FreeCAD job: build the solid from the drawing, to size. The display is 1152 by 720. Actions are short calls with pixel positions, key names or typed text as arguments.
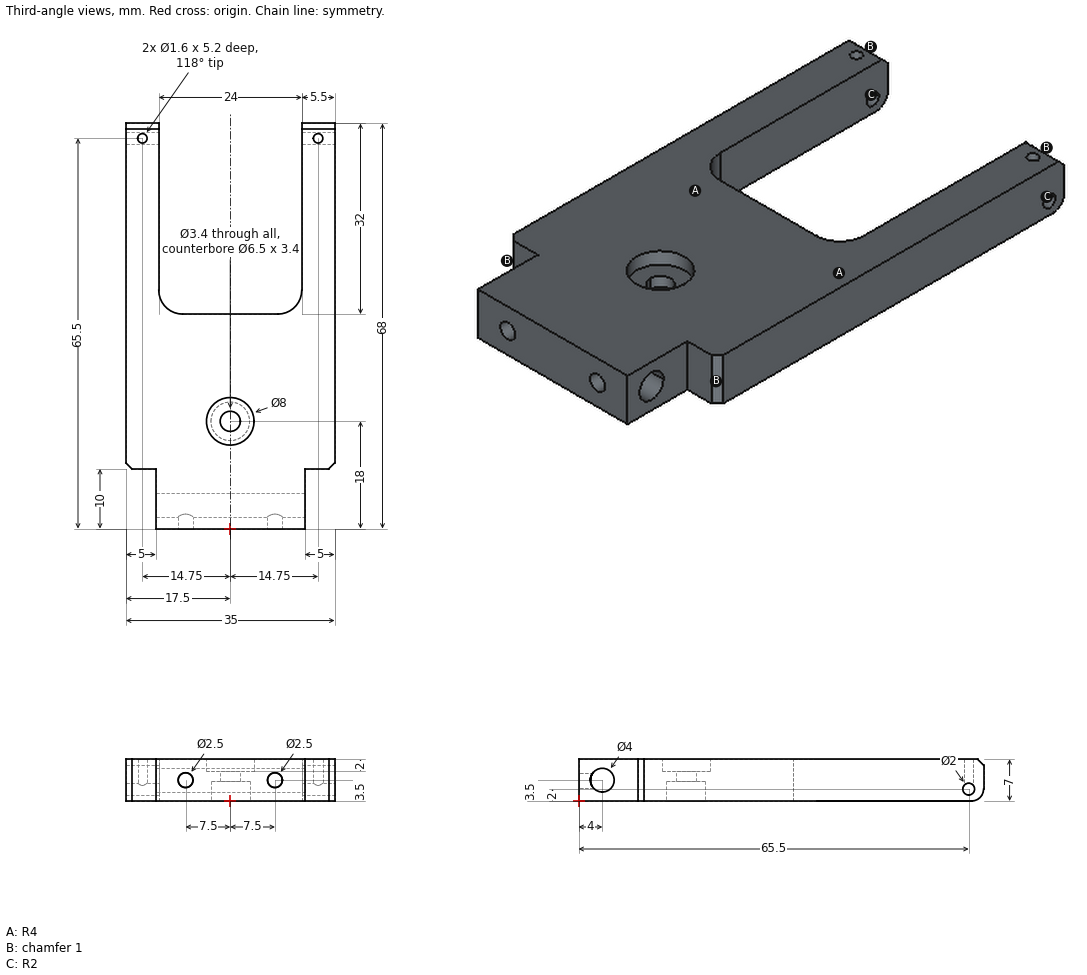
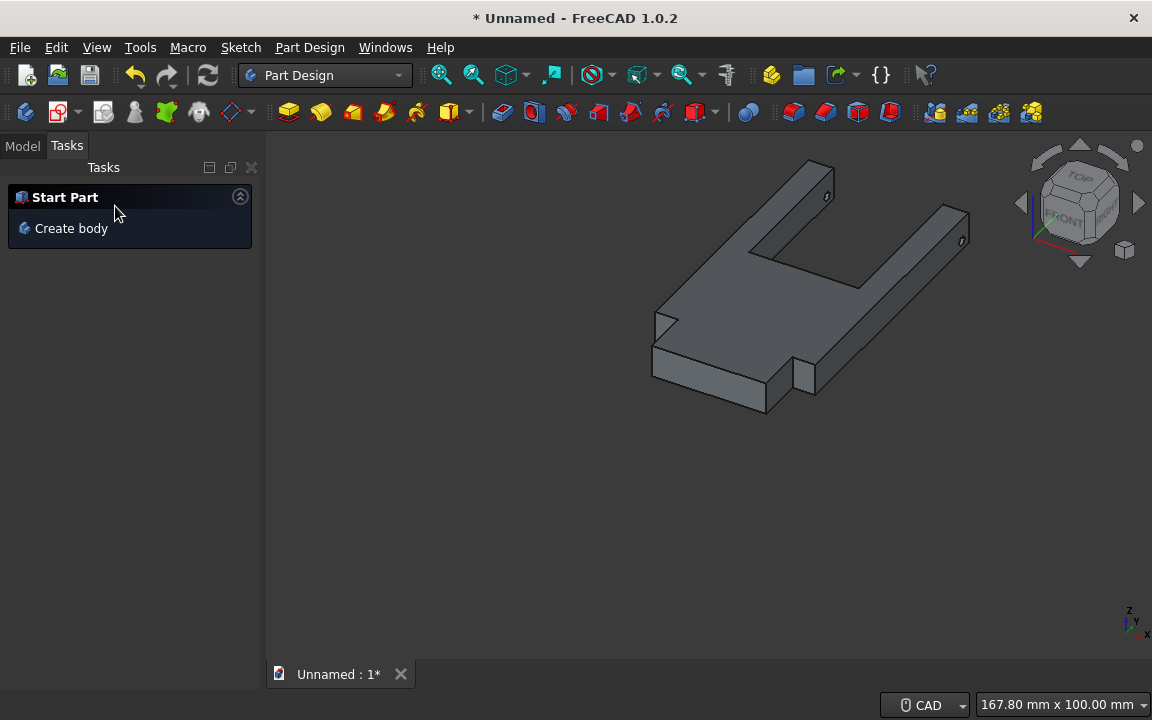
click(783, 381)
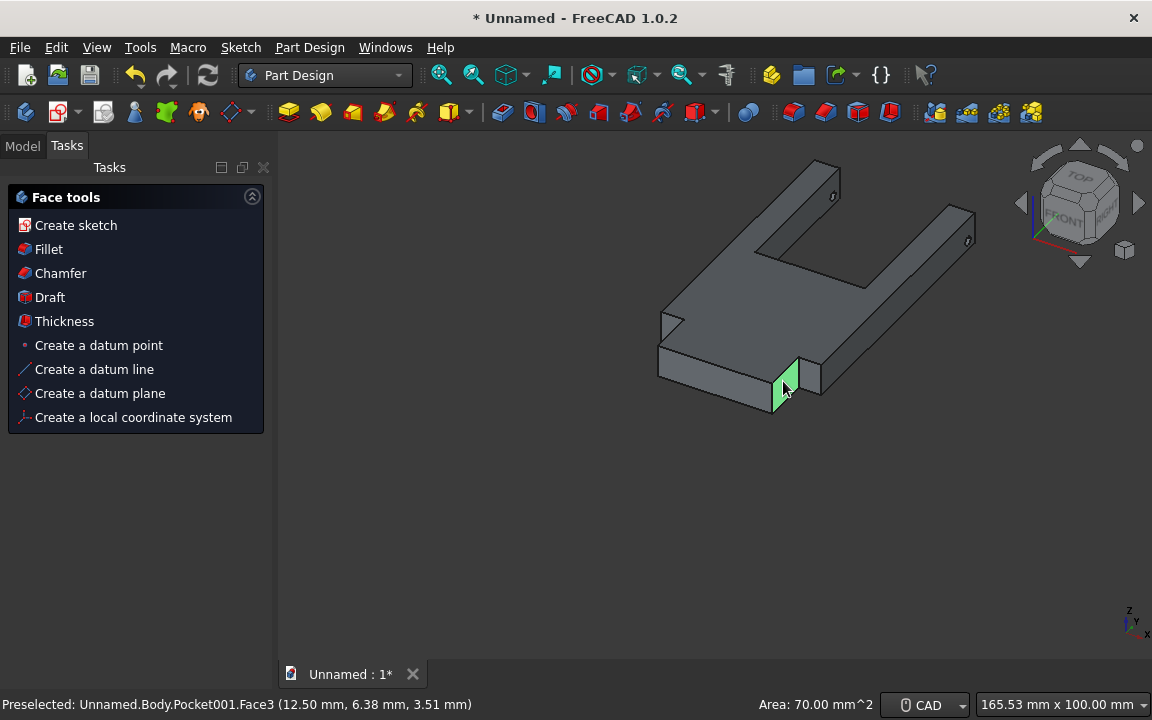
click(58, 112)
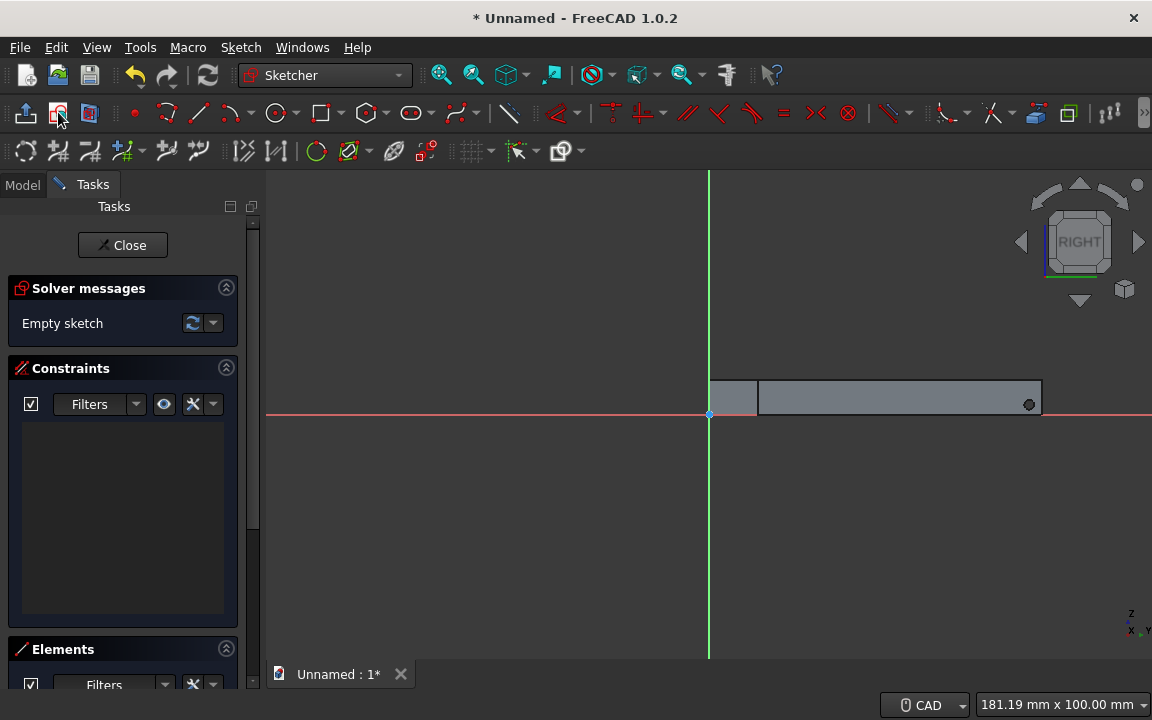
scroll(732, 400, up, 12)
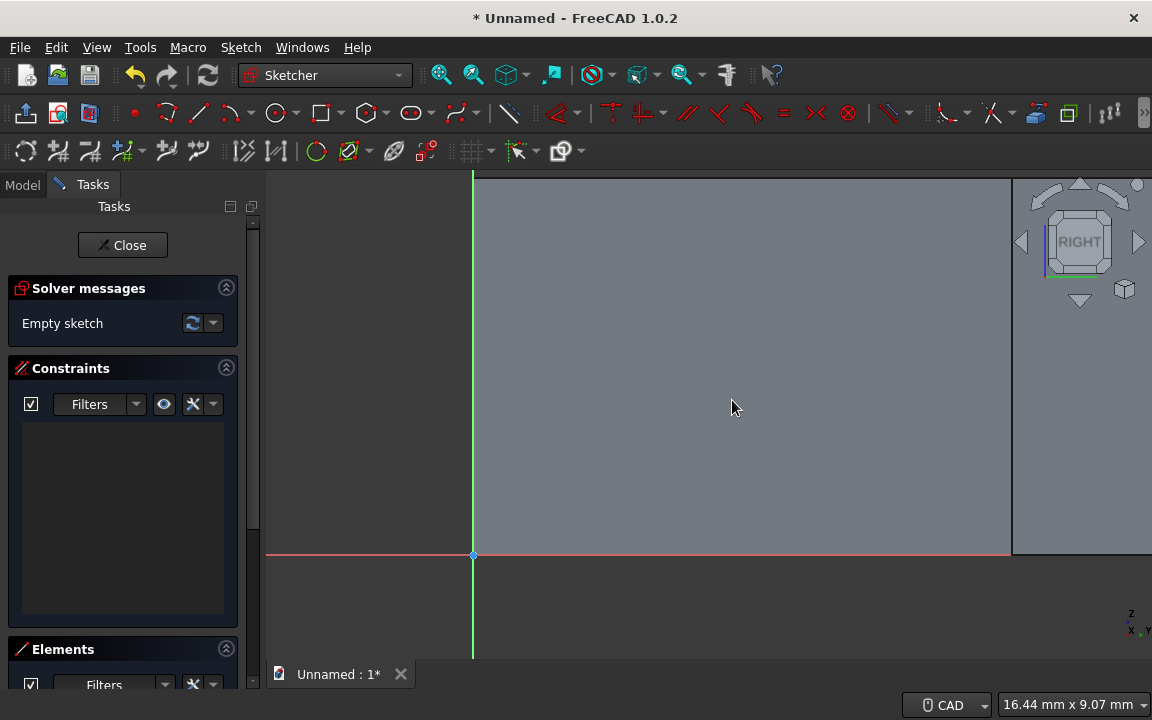
key(g)
key(c)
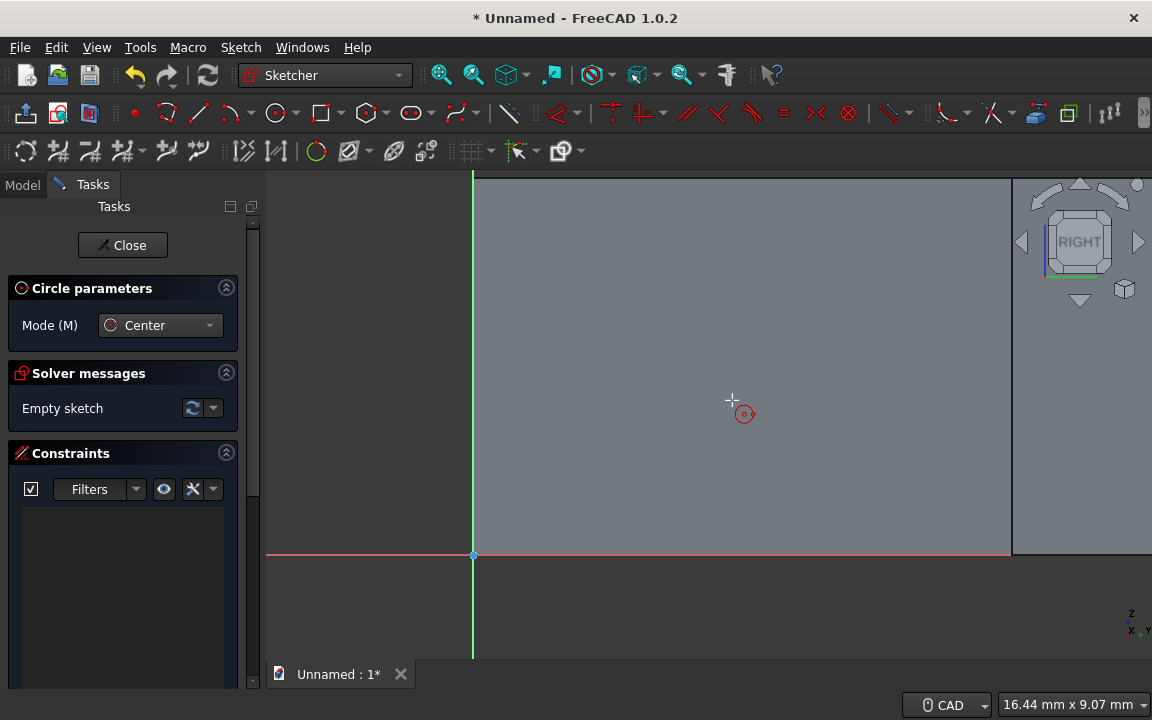
click(689, 366)
move(765, 290)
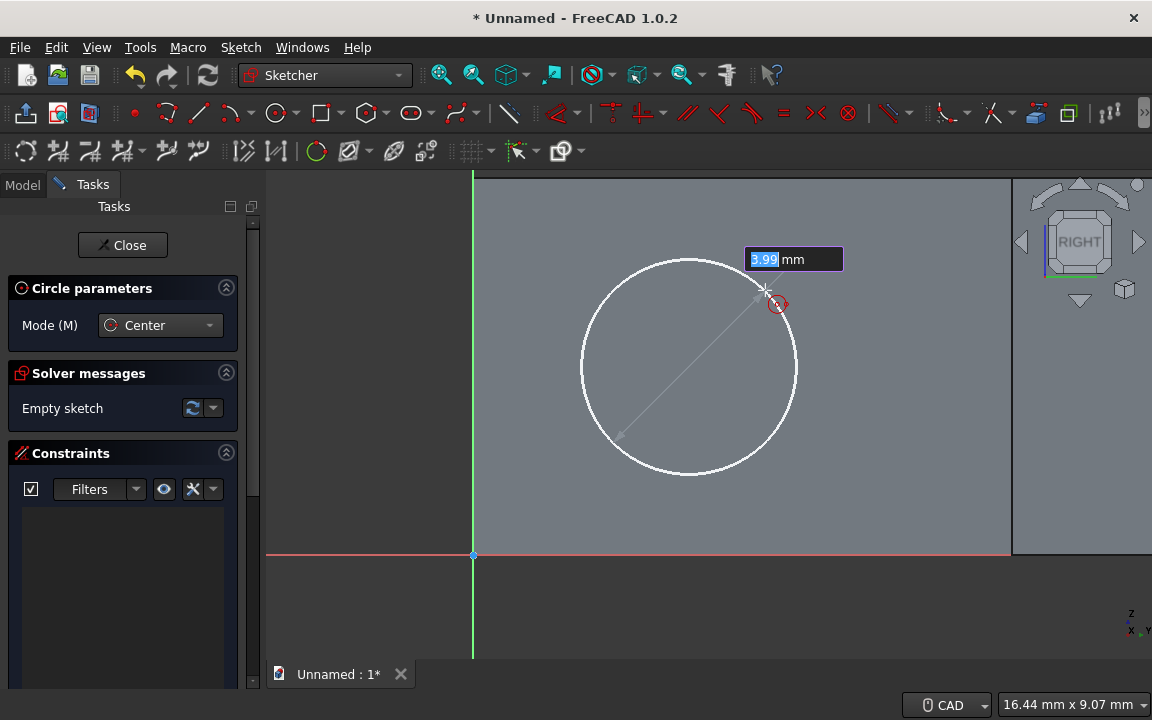
text(4)
key(Return)
key(Escape)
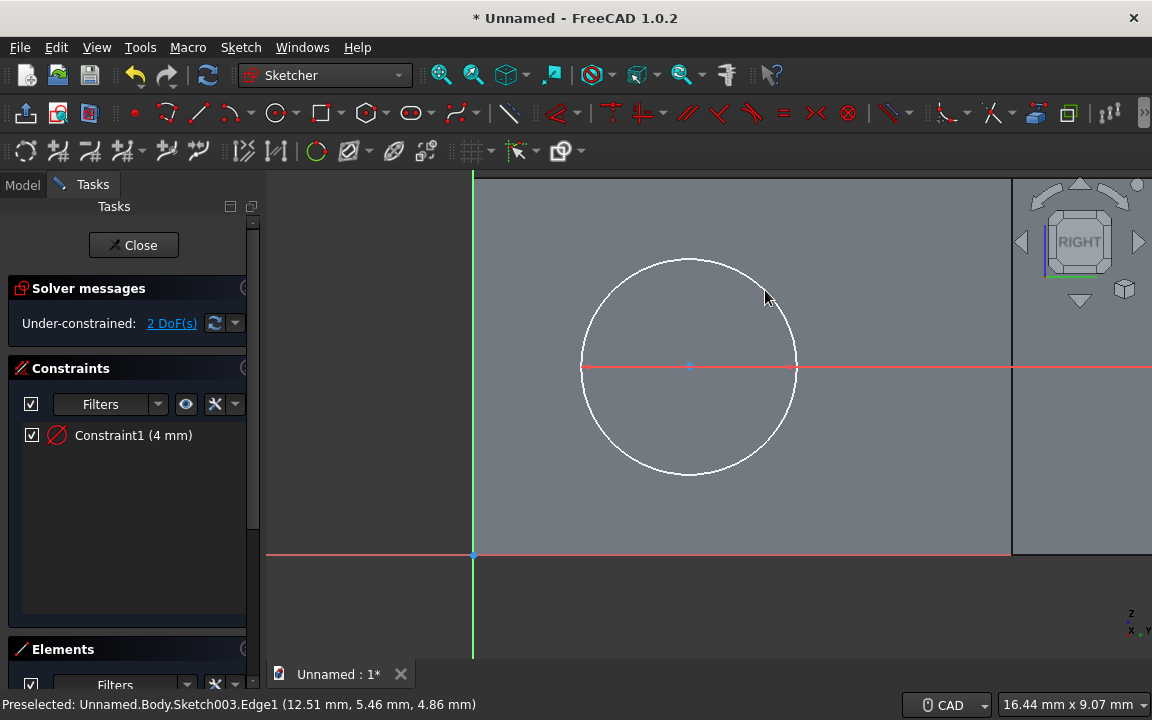
key(d)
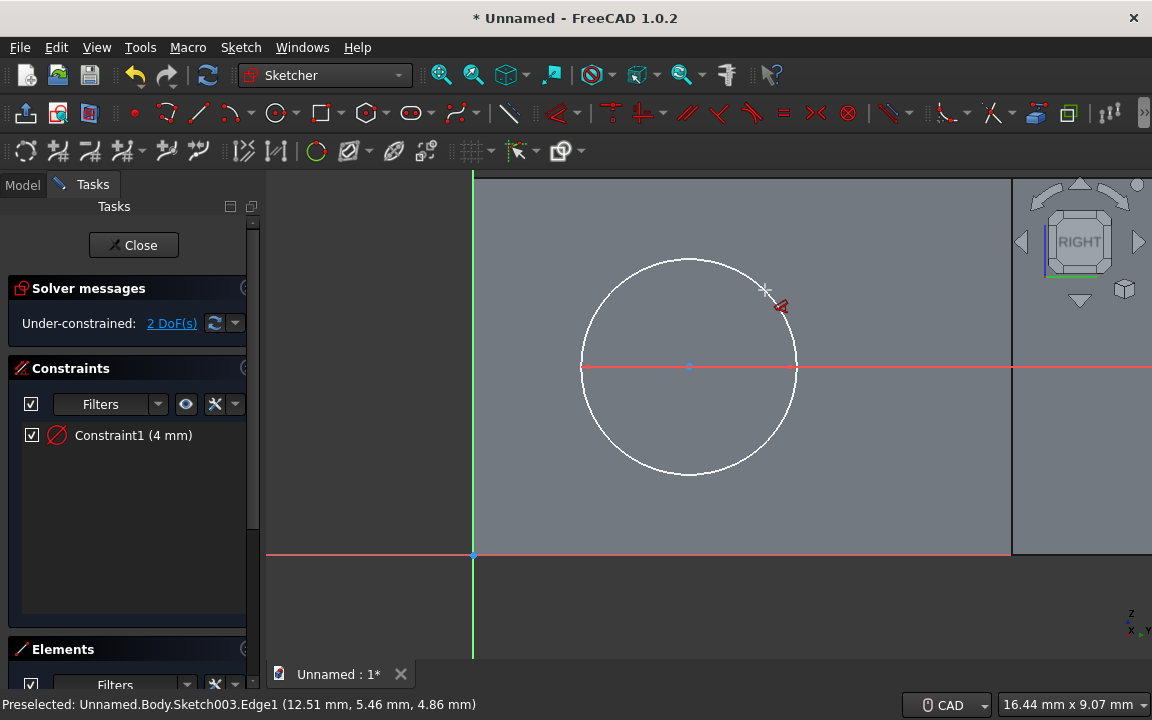
click(689, 367)
click(581, 589)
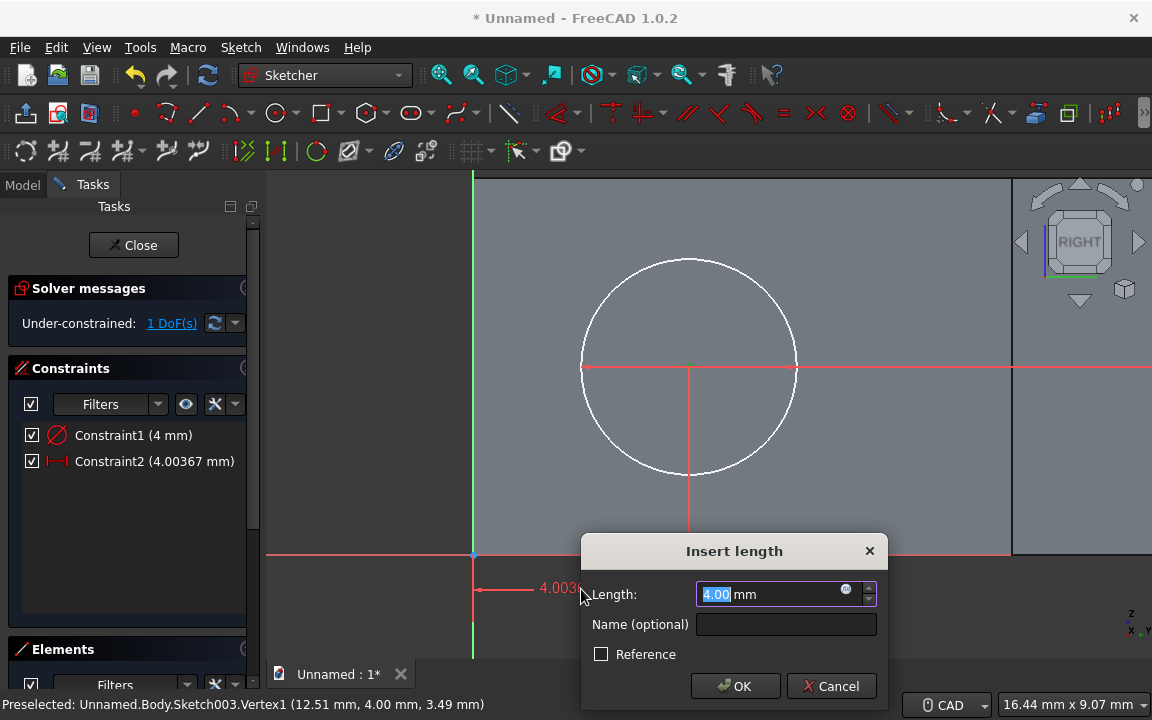
text(4)
key(Return)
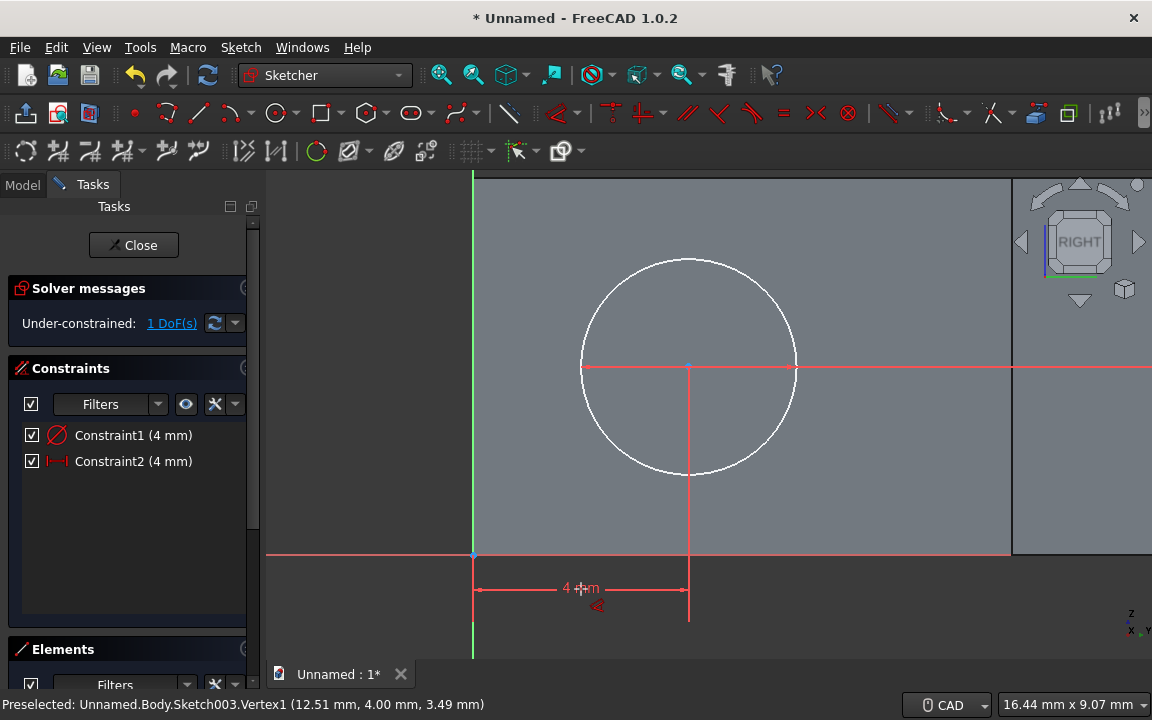
click(689, 367)
click(439, 461)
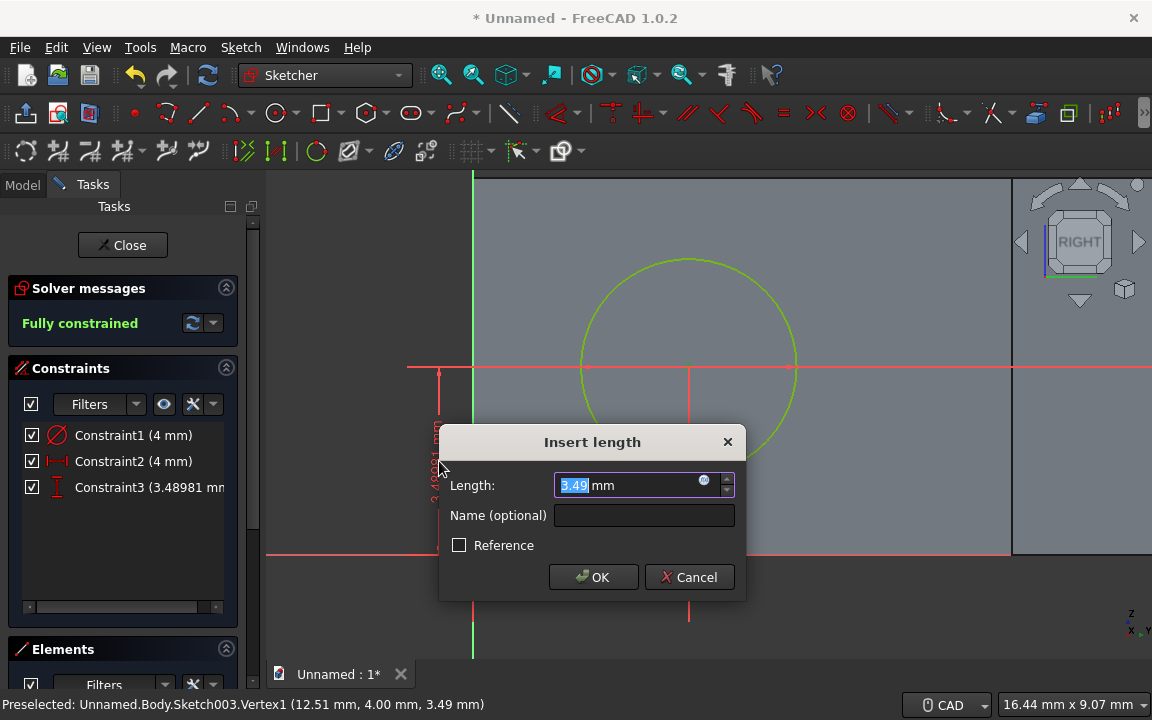
text(3.5)
key(Return)
key(Escape)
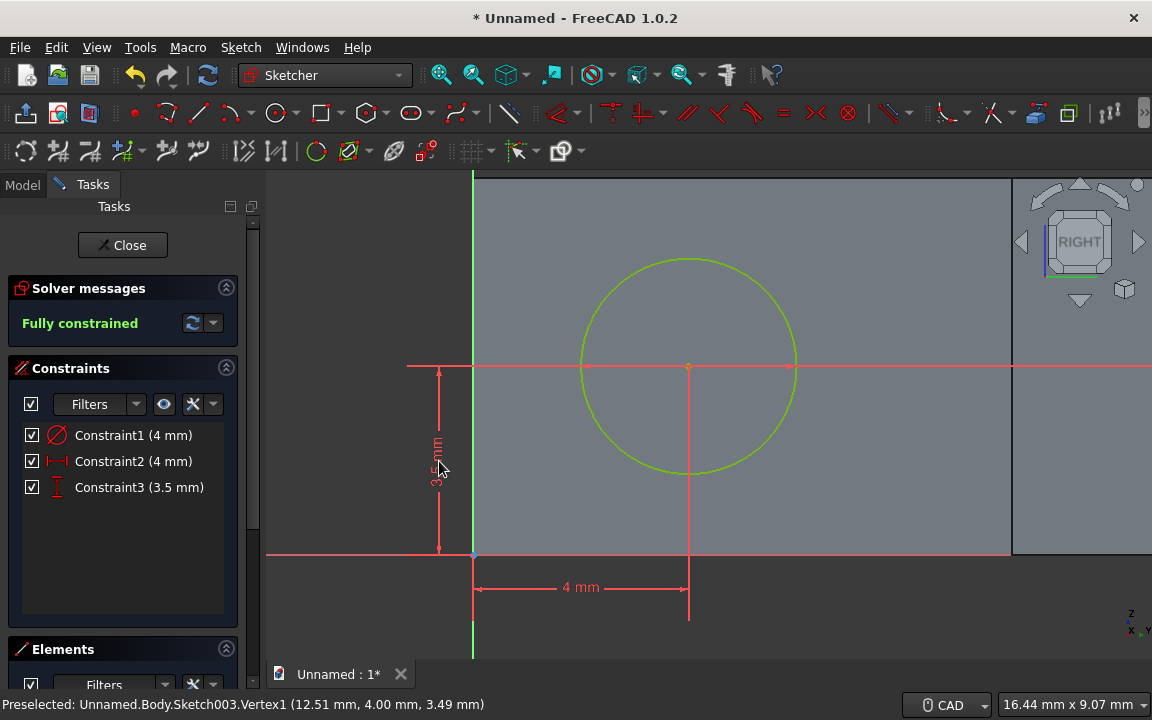
click(123, 245)